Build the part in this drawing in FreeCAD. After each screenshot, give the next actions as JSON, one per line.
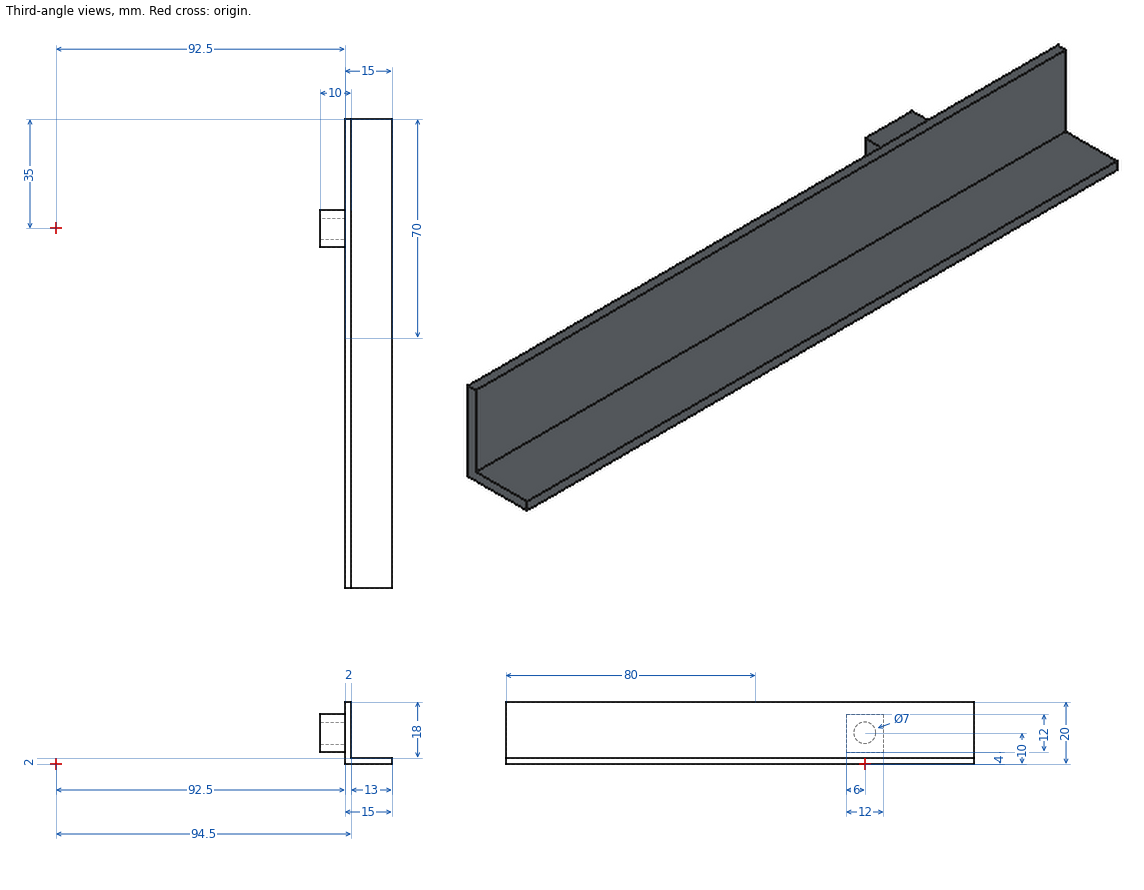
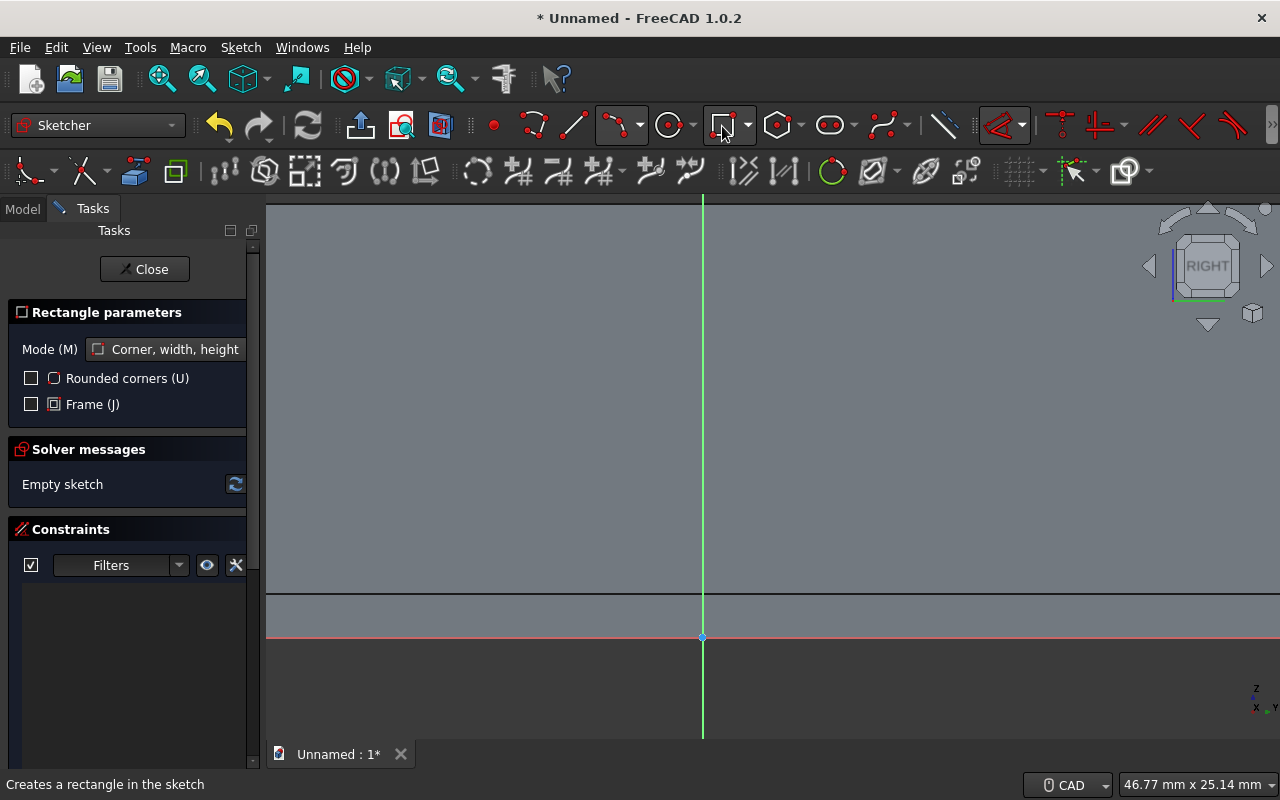
{"action": "left_click", "coordinate": [573, 291]}
{"action": "left_click", "coordinate": [833, 551]}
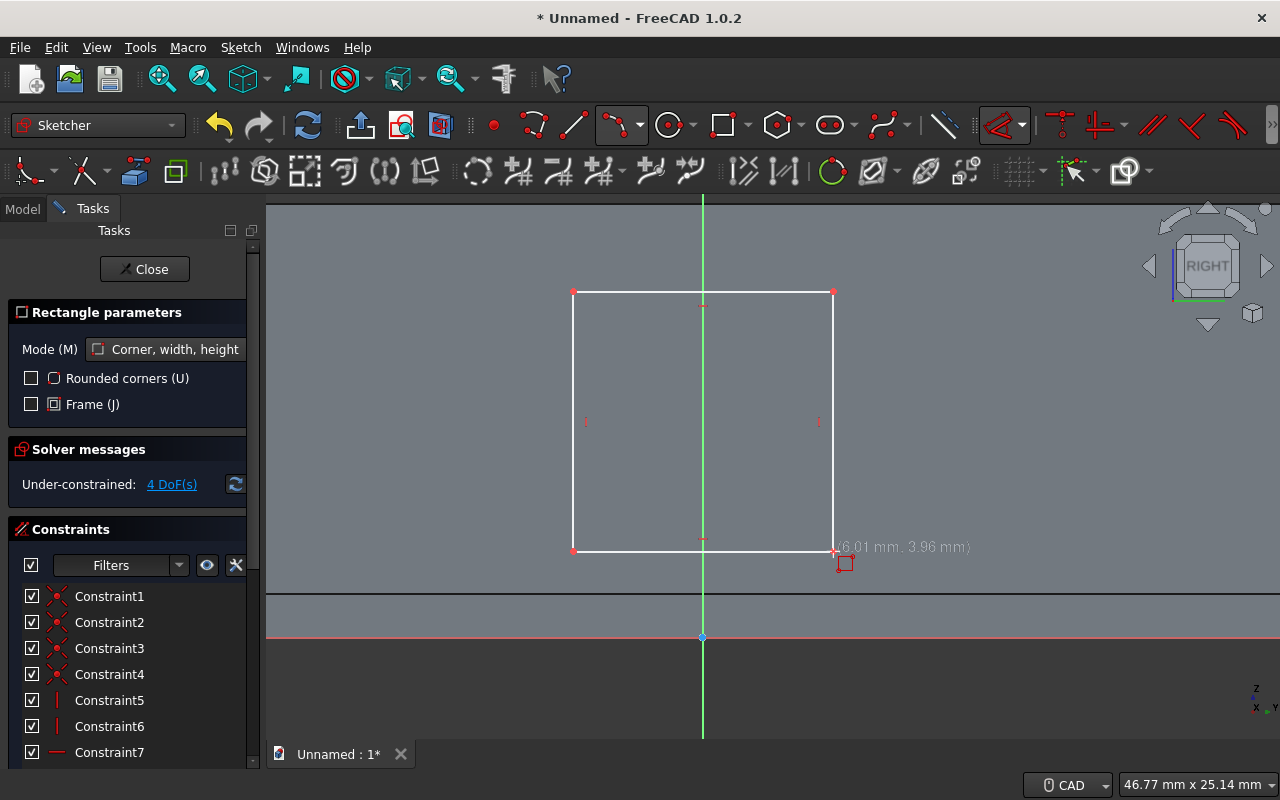
{"action": "left_click", "coordinate": [670, 126]}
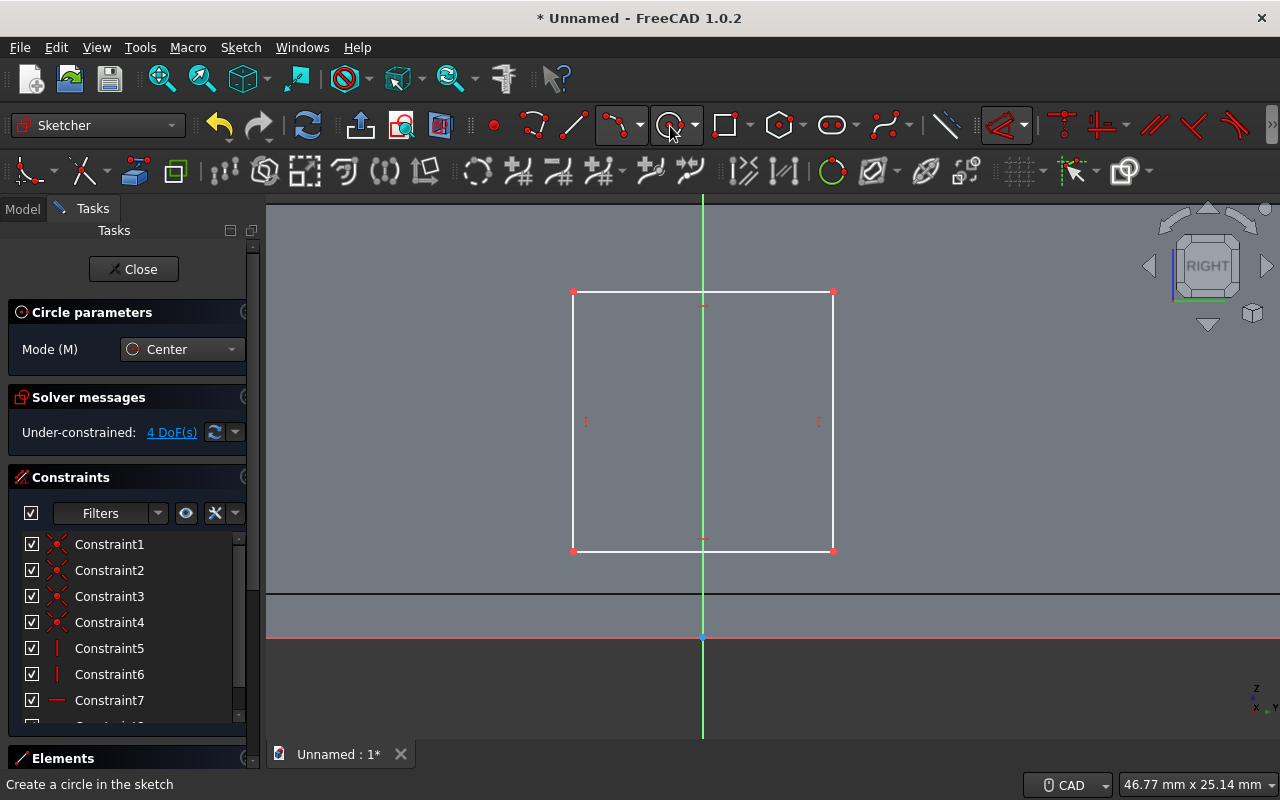
{"action": "left_click", "coordinate": [703, 421]}
{"action": "left_click", "coordinate": [756, 367]}
{"action": "key", "text": "Escape"}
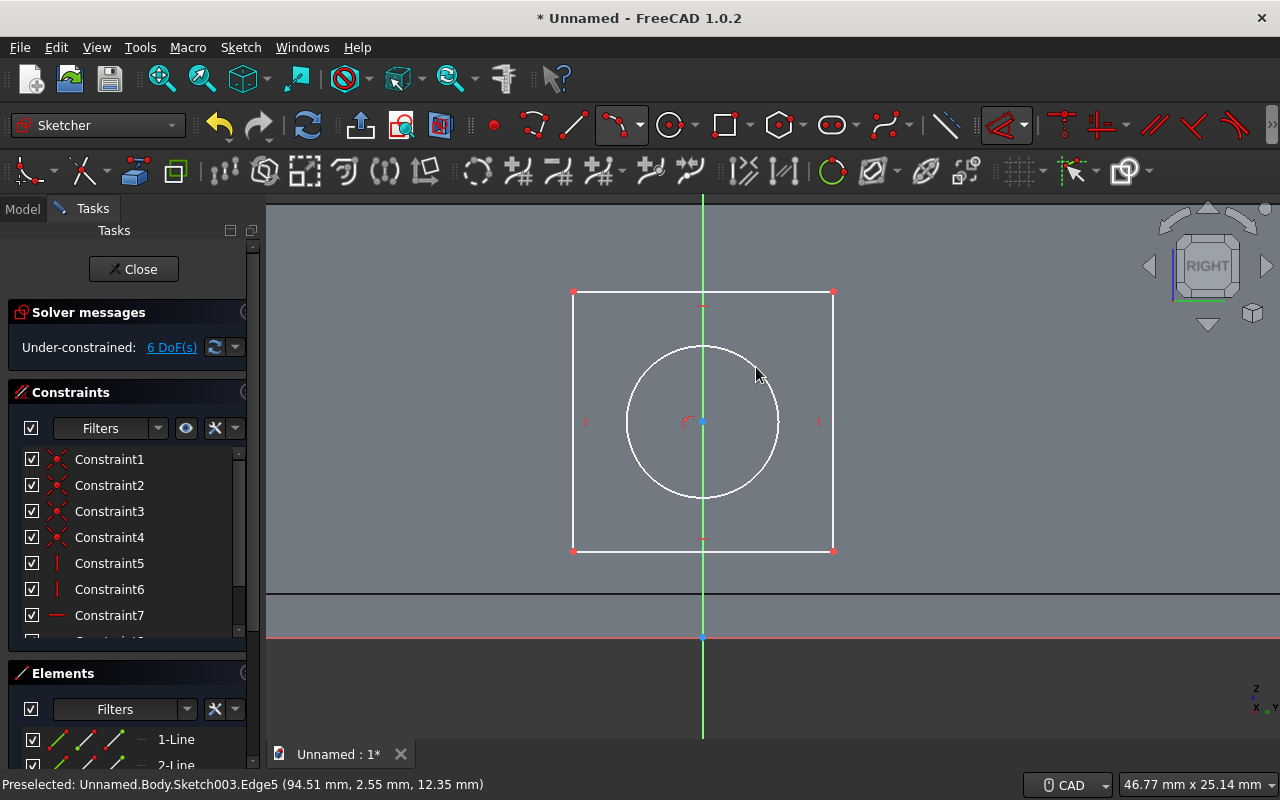
{"action": "left_click", "coordinate": [756, 368]}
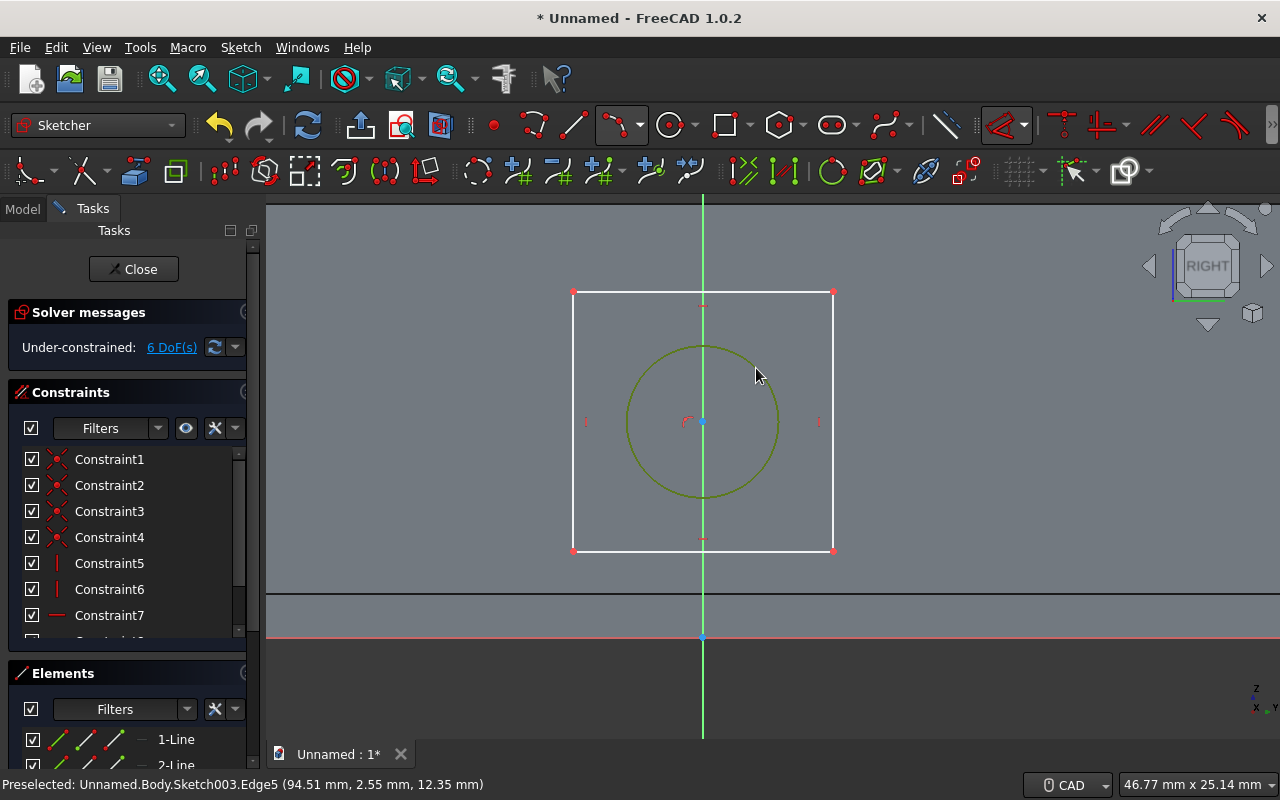
{"action": "key", "text": "k o"}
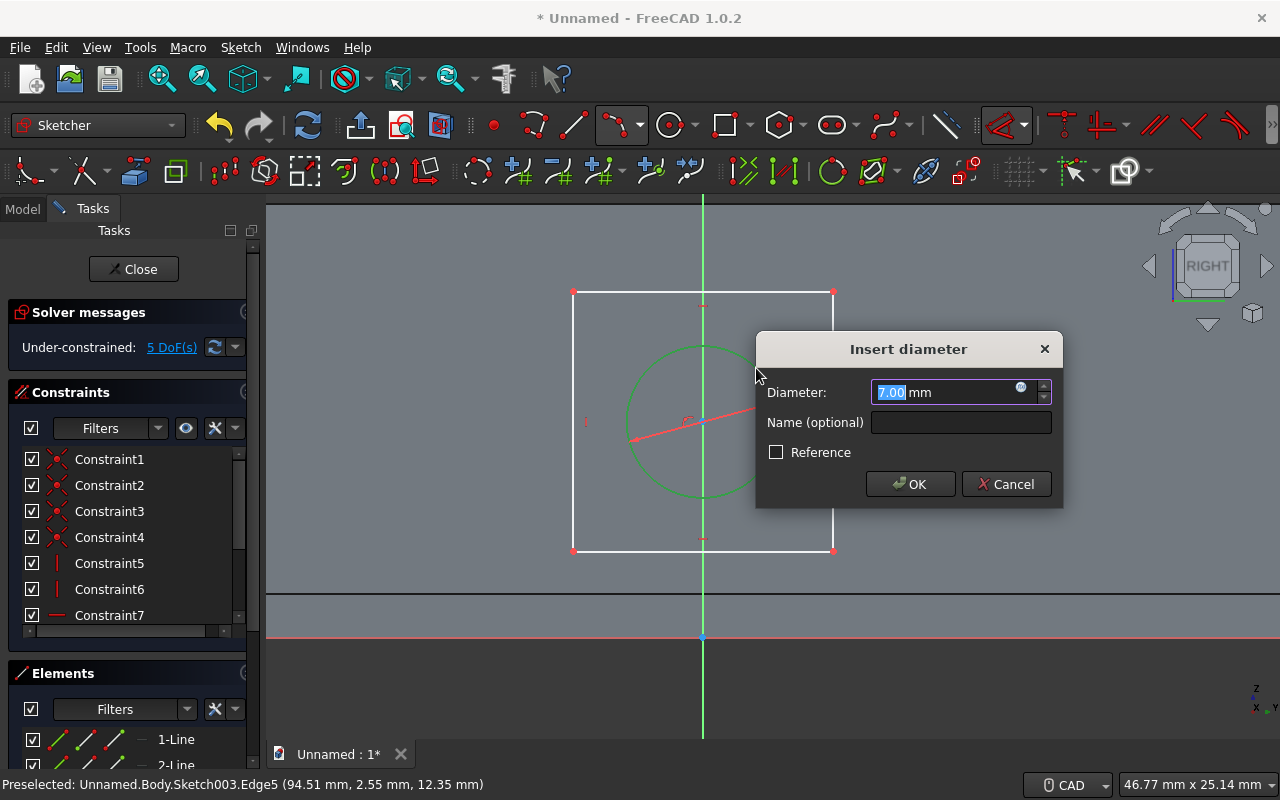
{"action": "type", "text": "7"}
{"action": "key", "text": "Return"}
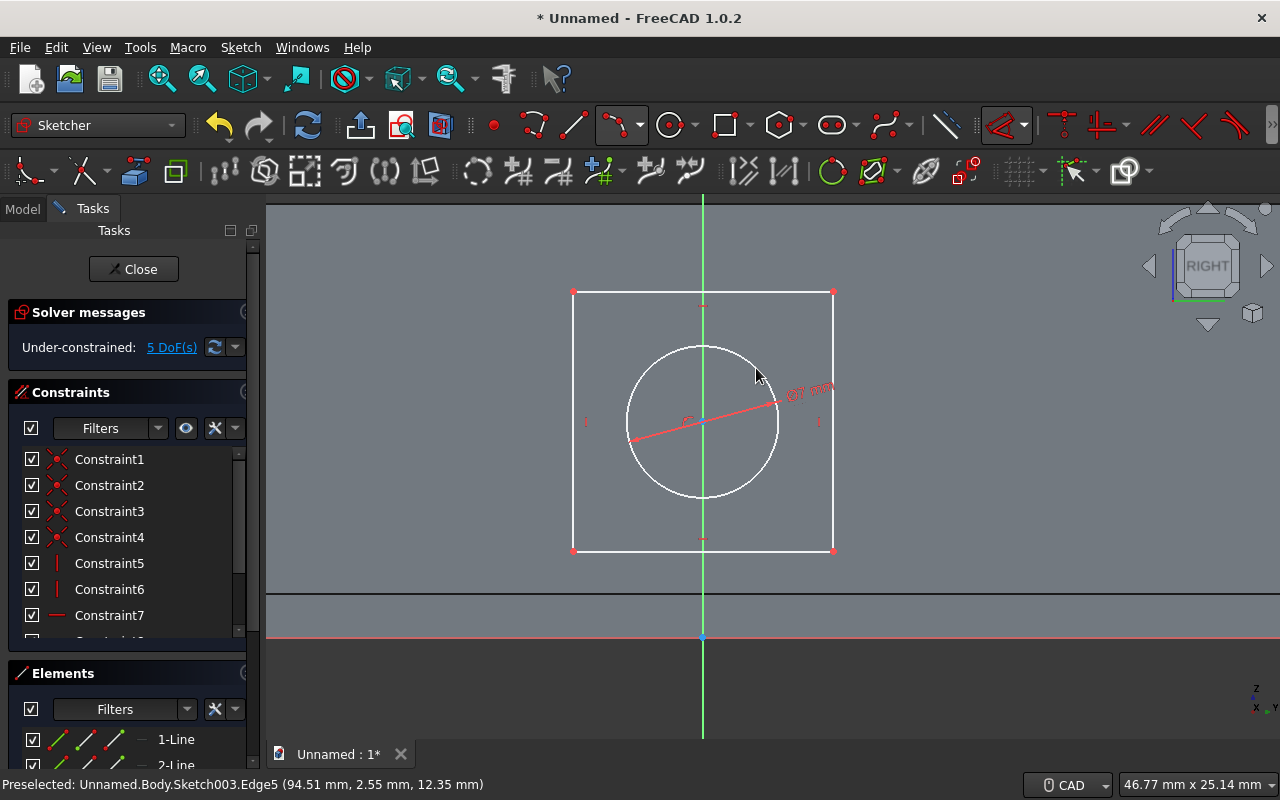
{"action": "left_click", "coordinate": [573, 370]}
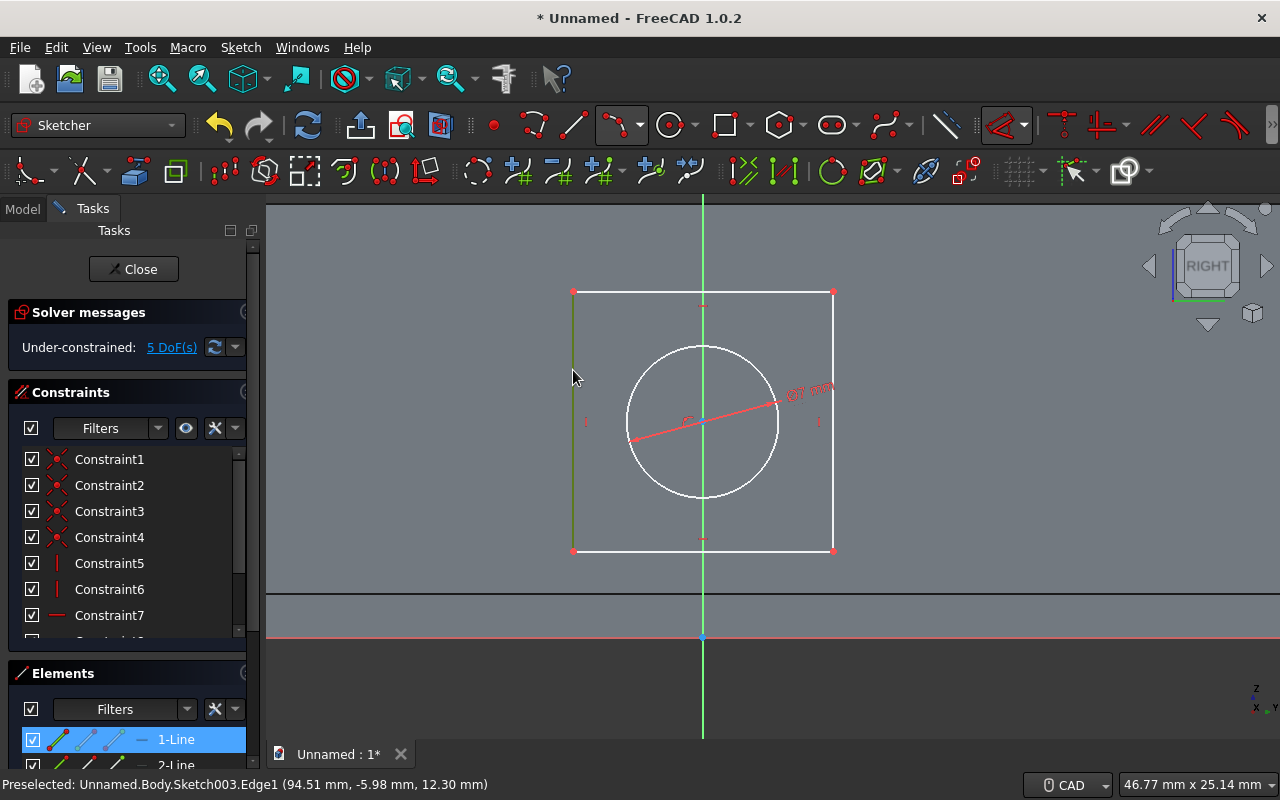
{"action": "left_click", "coordinate": [1026, 126]}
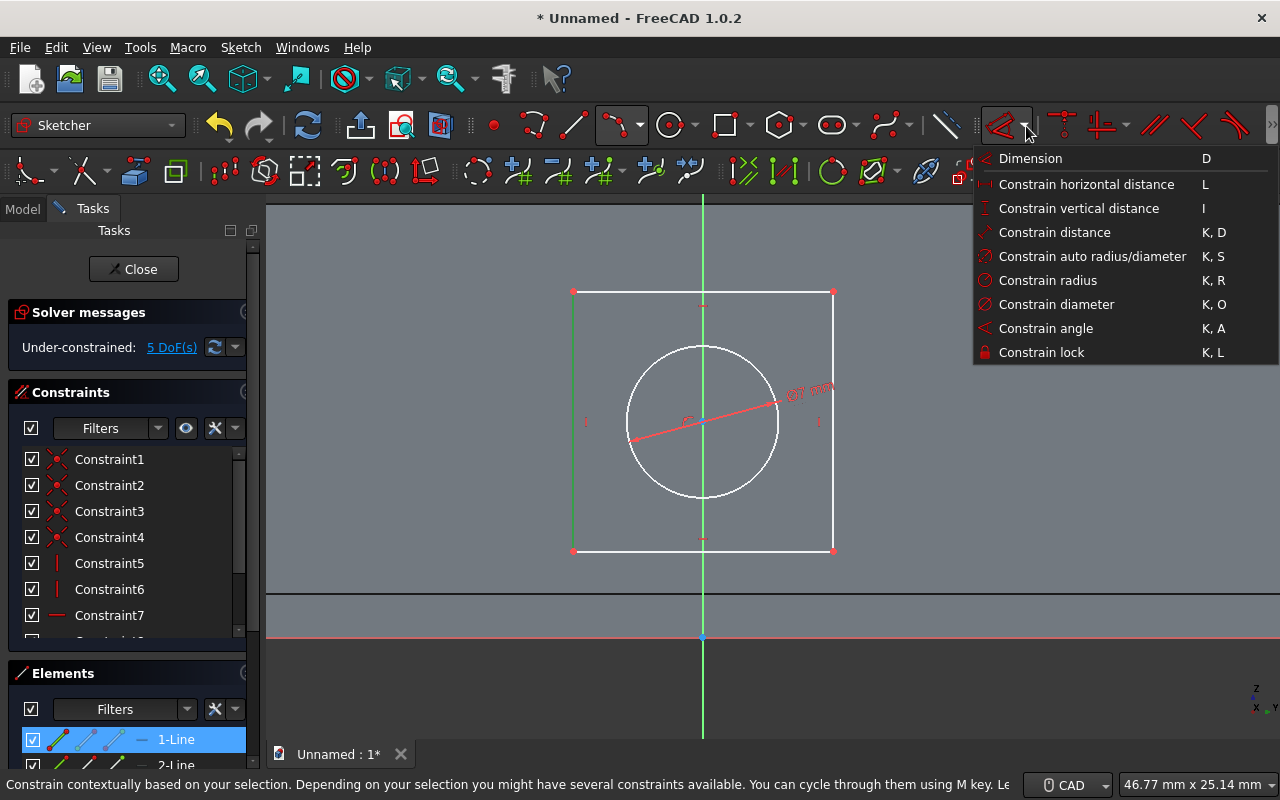
{"action": "left_click", "coordinate": [1126, 208]}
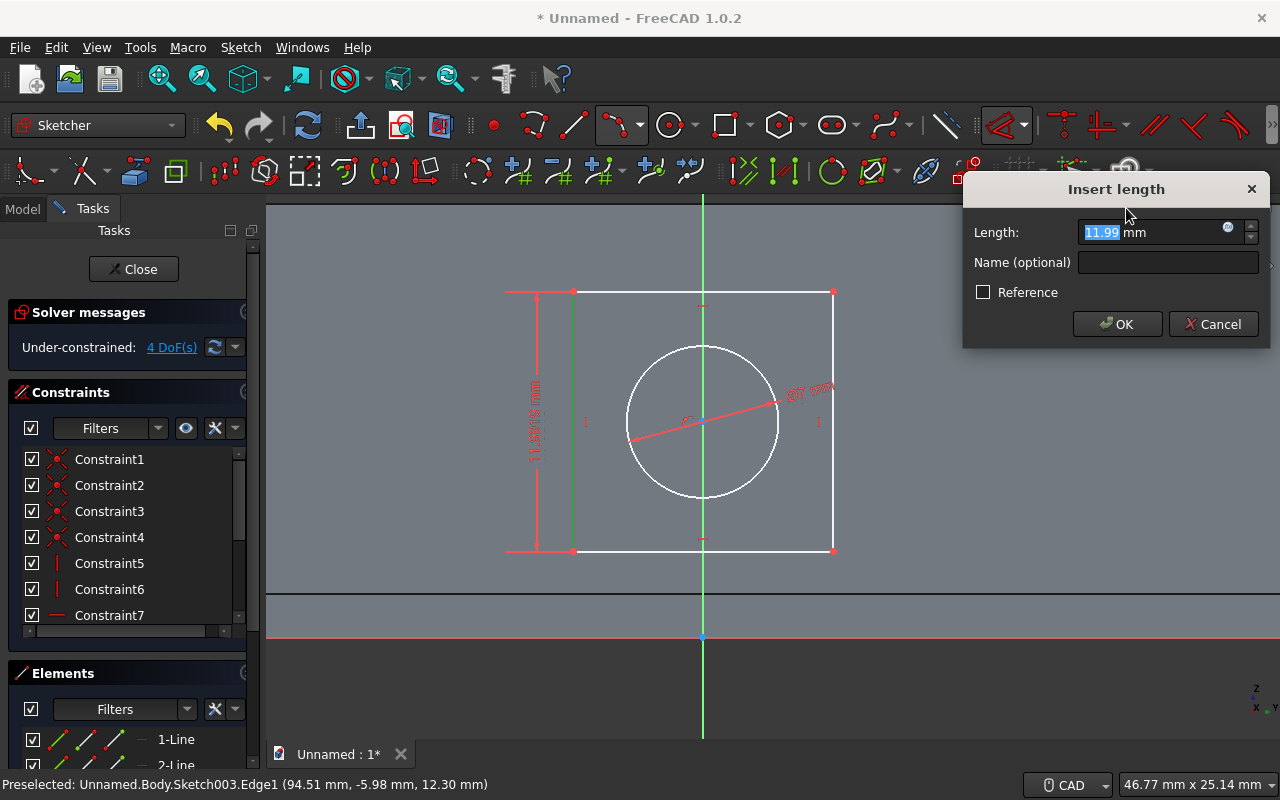
{"action": "type", "text": "12"}
{"action": "key", "text": "Return"}